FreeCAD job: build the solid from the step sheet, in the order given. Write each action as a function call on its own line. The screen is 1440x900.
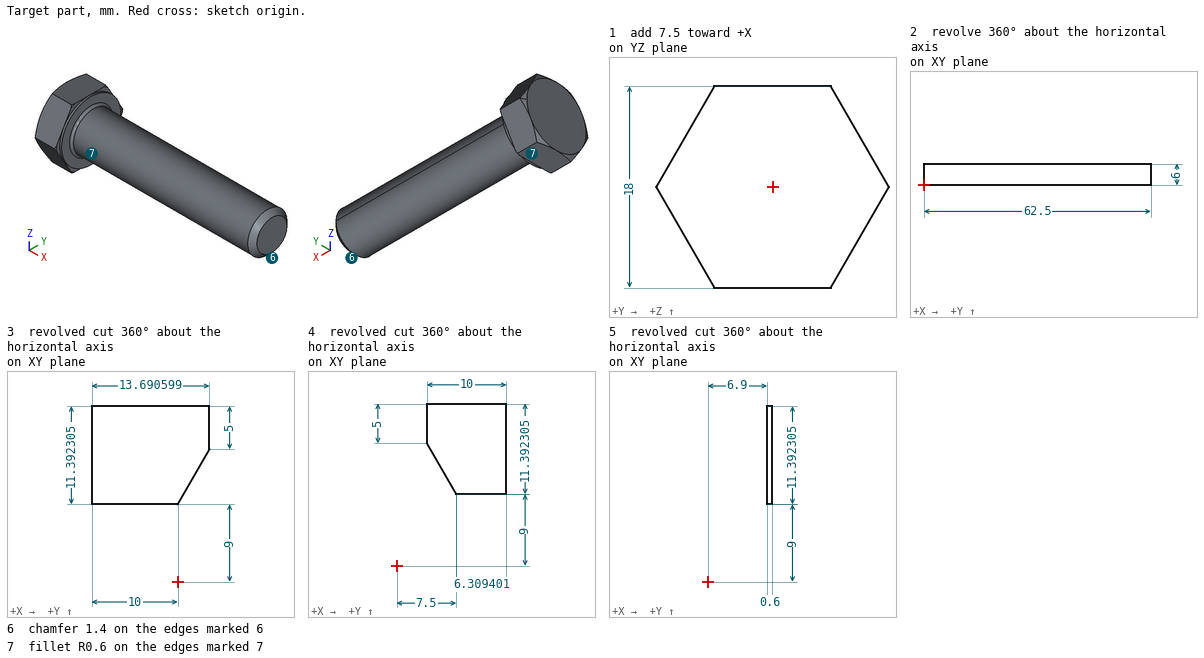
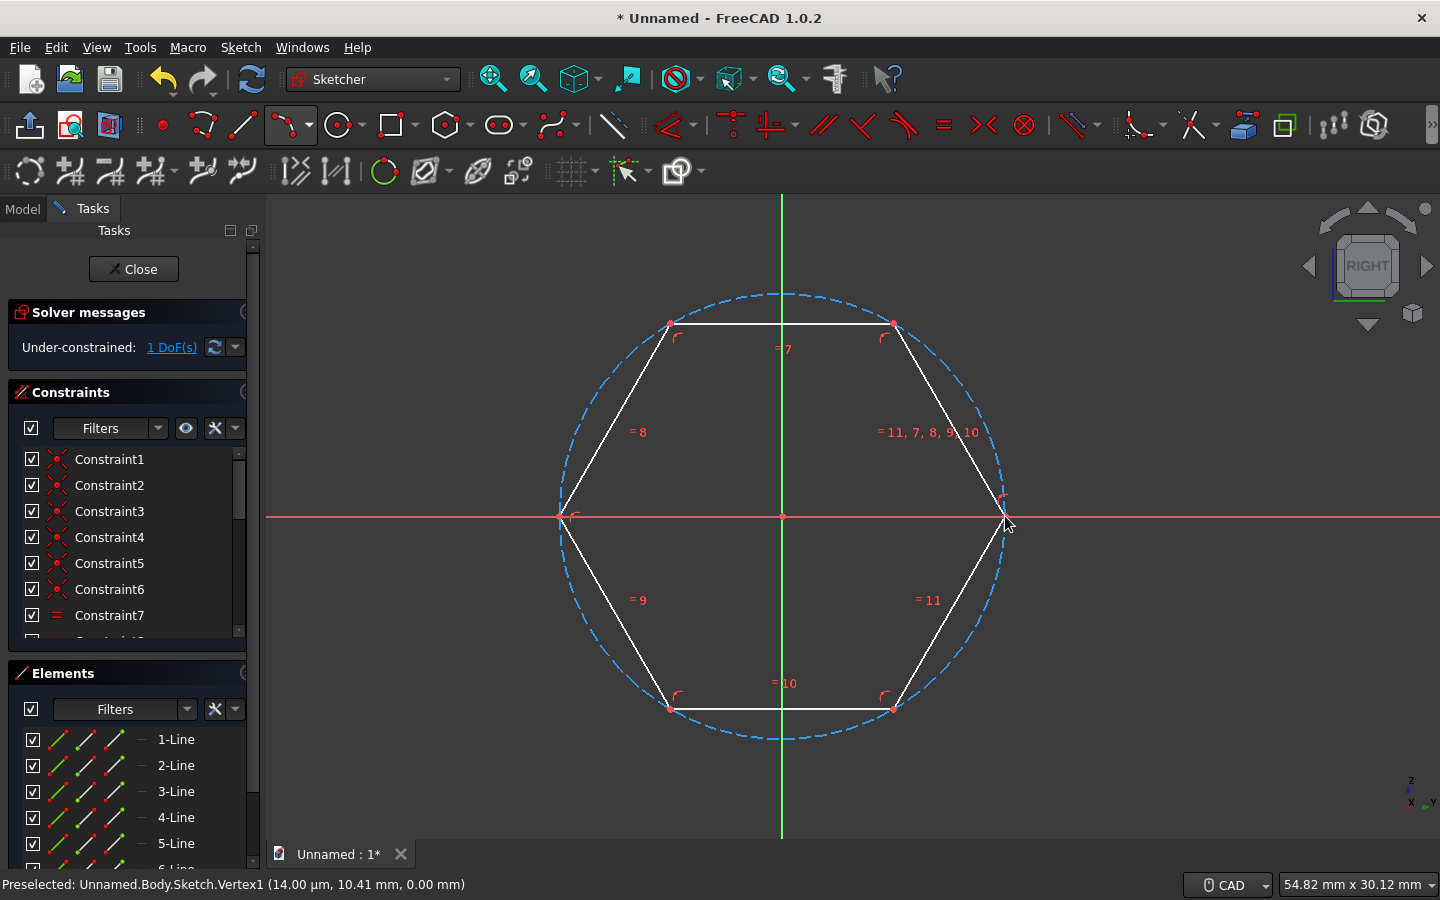
click(668, 126)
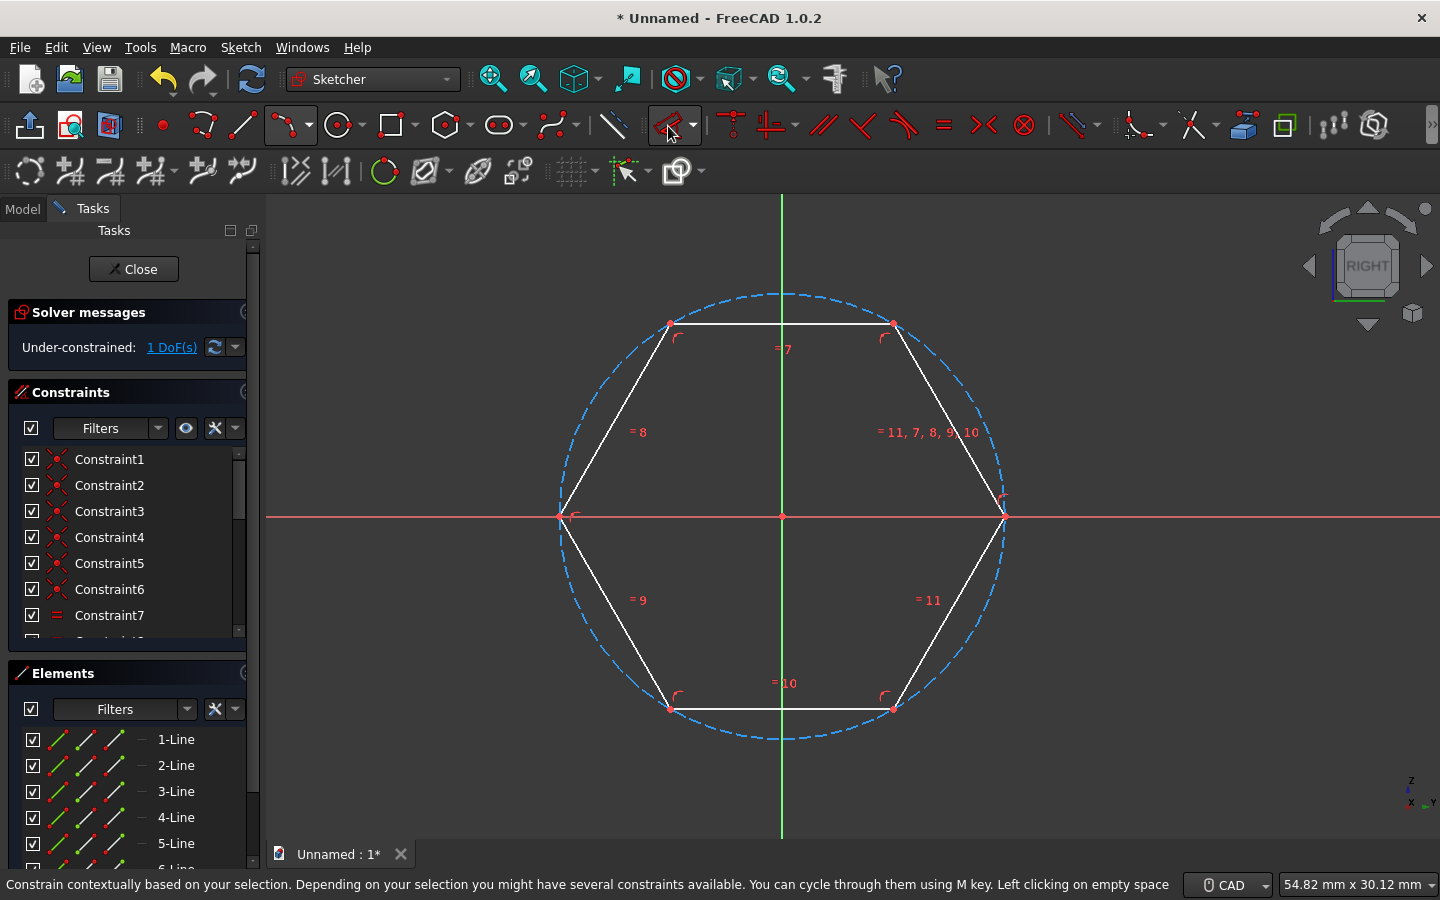
click(671, 709)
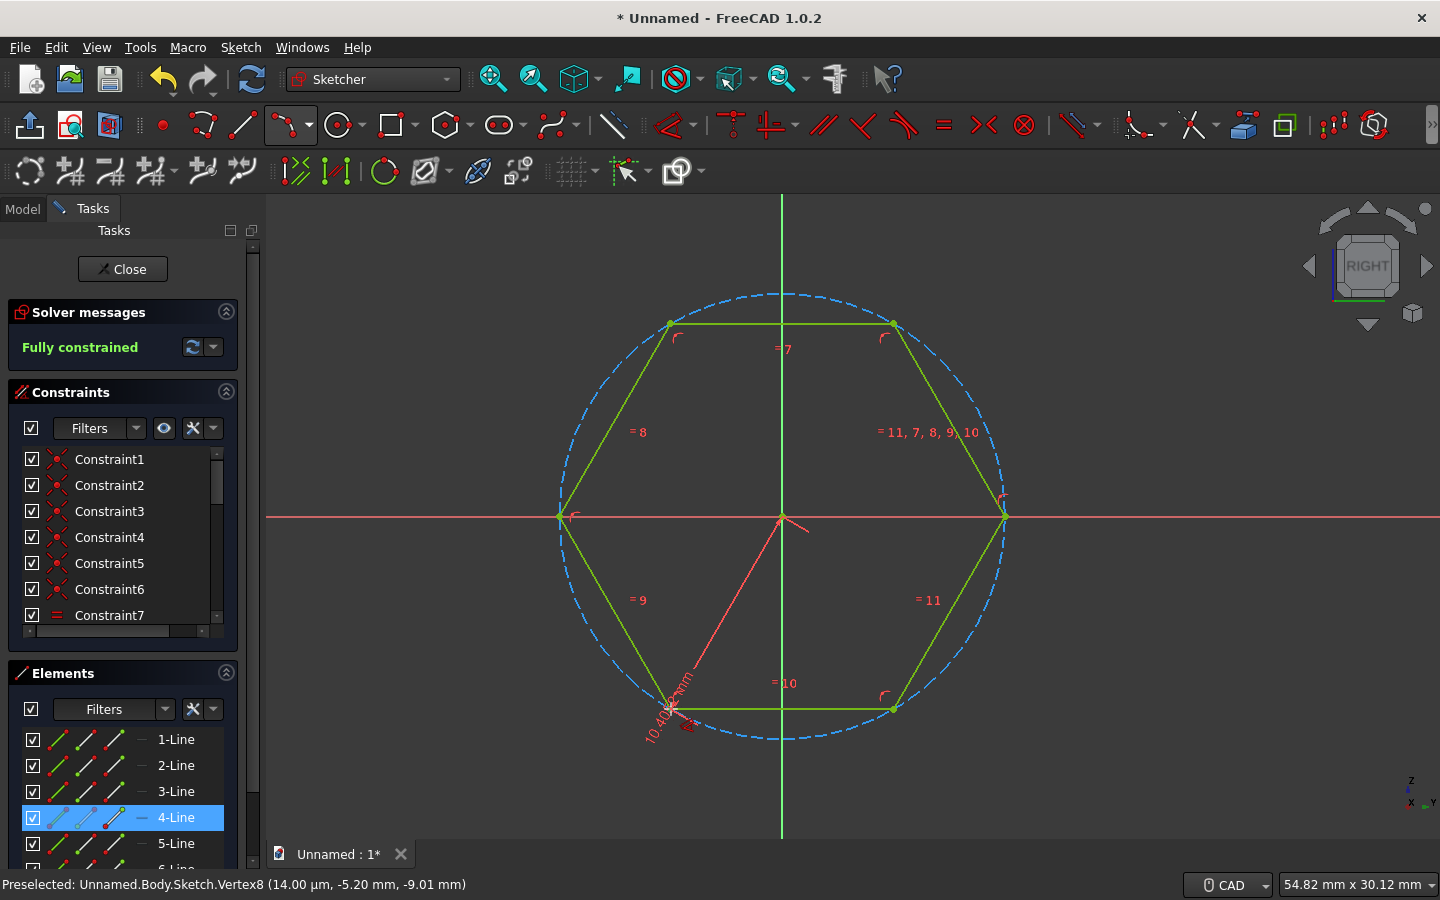
click(894, 324)
click(928, 428)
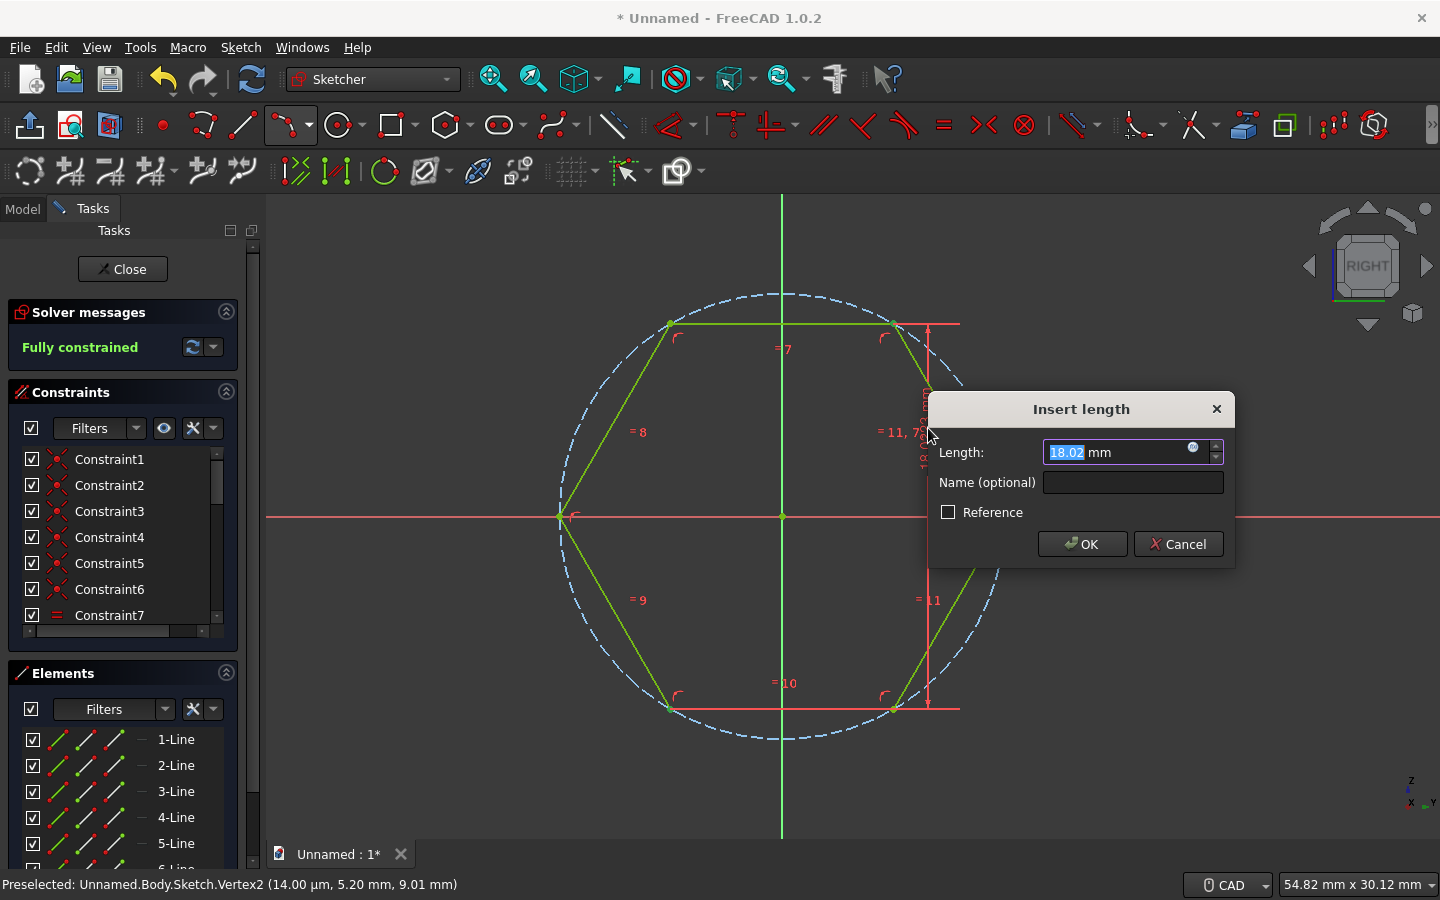
text(18)
key(Return)
key(Escape)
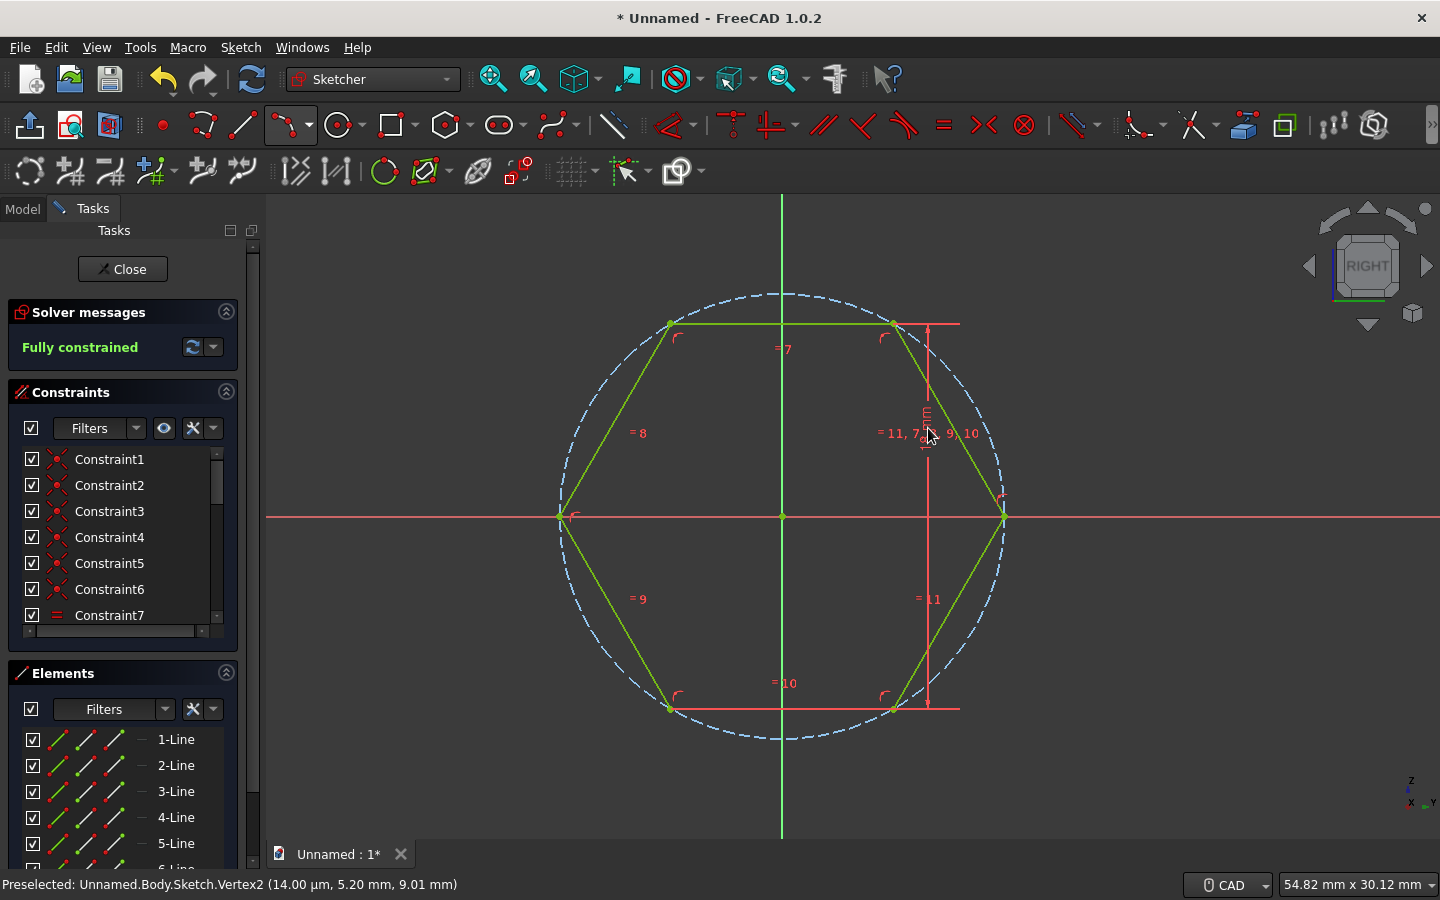
click(123, 269)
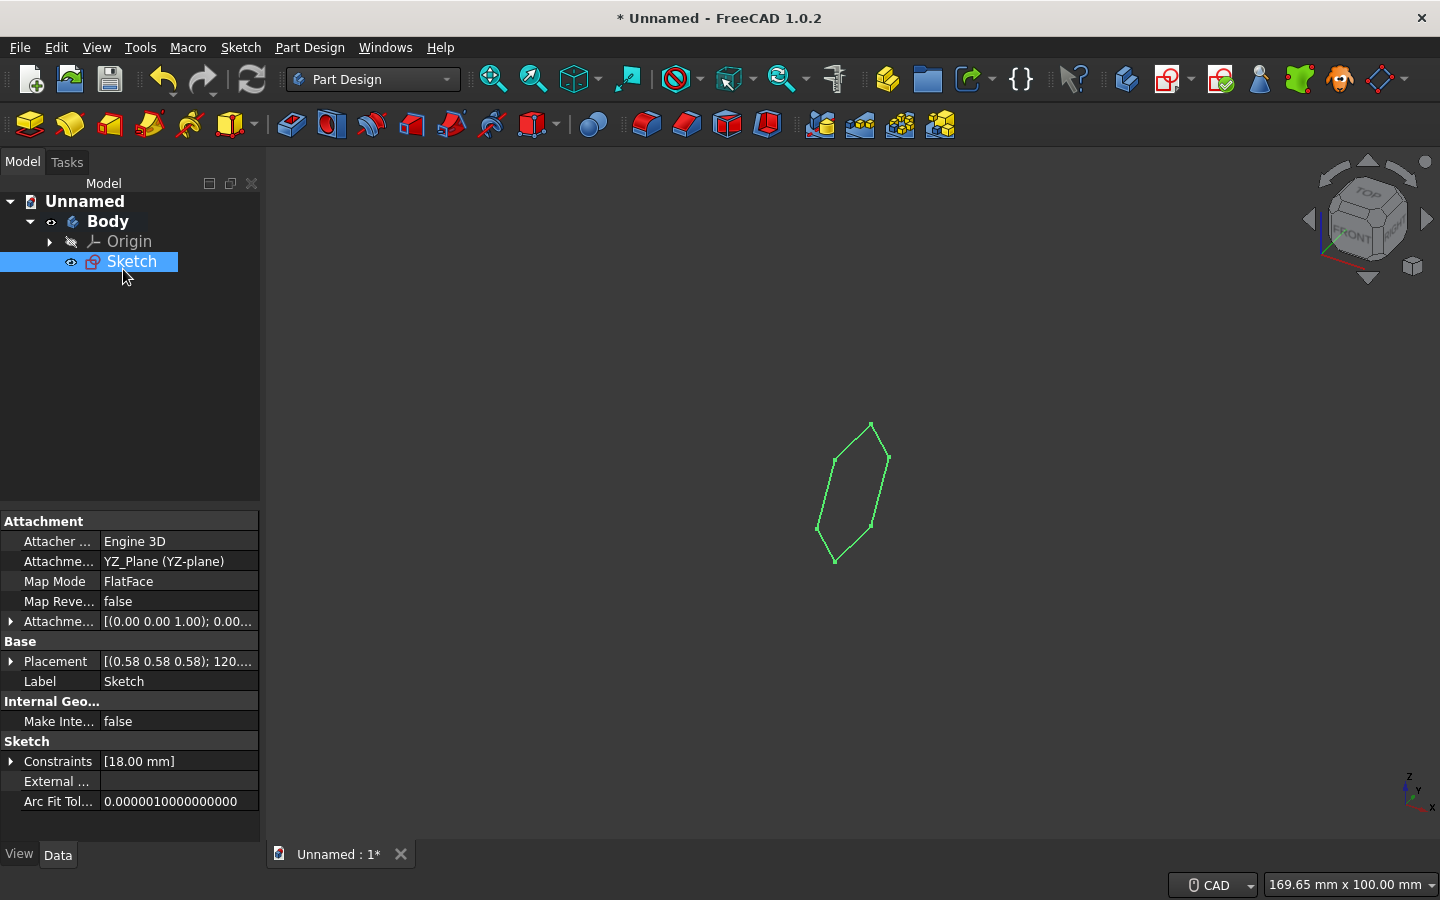
click(30, 124)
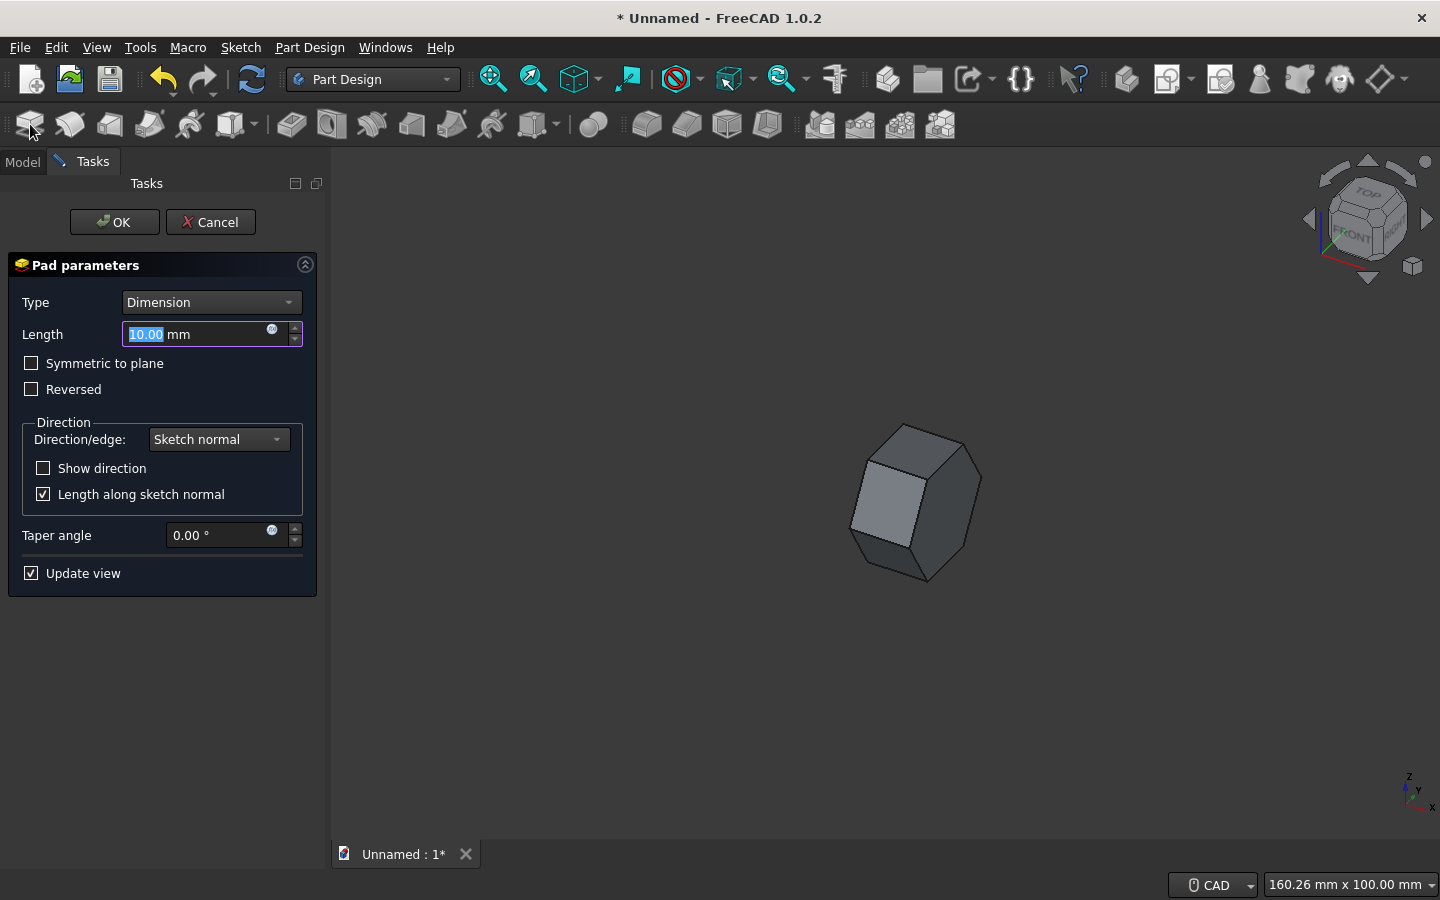
text(7.5)
key(Tab)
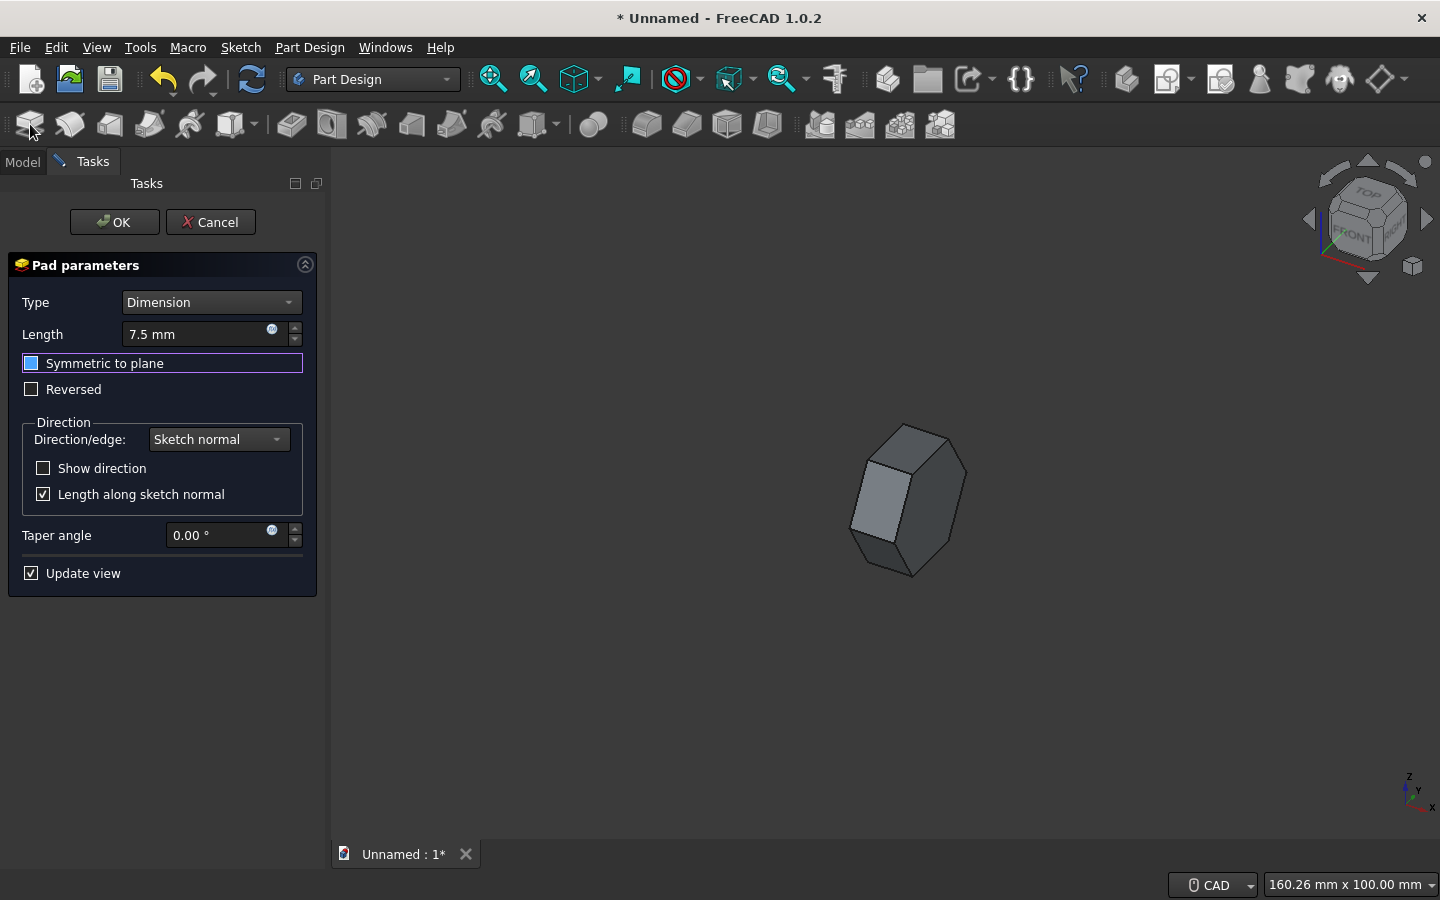
click(115, 222)